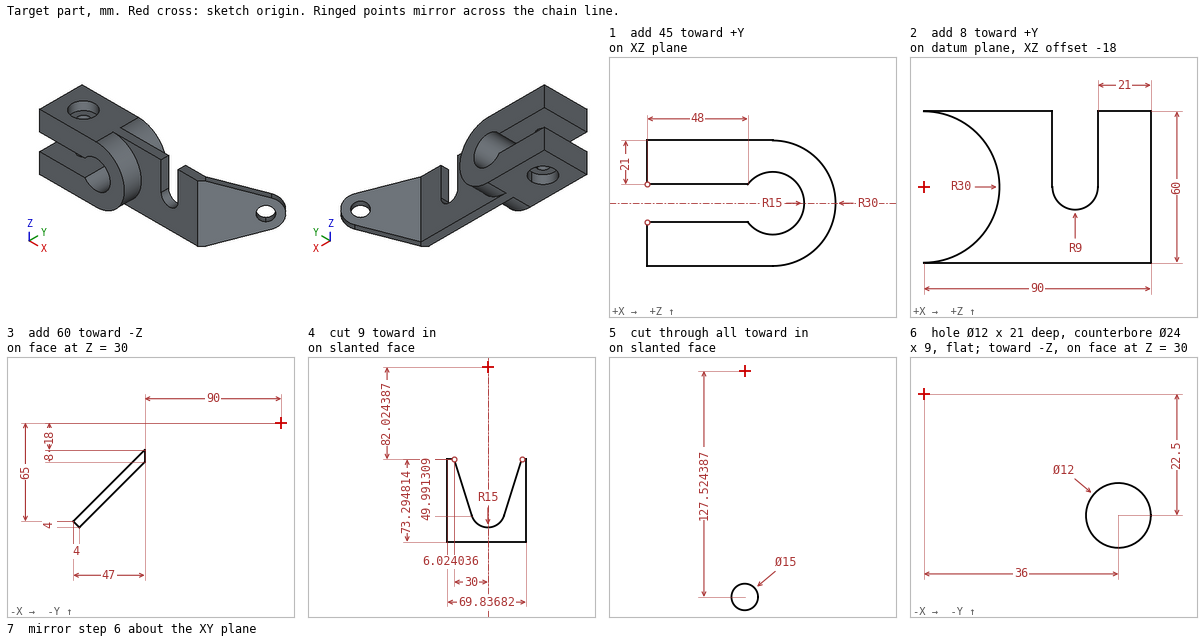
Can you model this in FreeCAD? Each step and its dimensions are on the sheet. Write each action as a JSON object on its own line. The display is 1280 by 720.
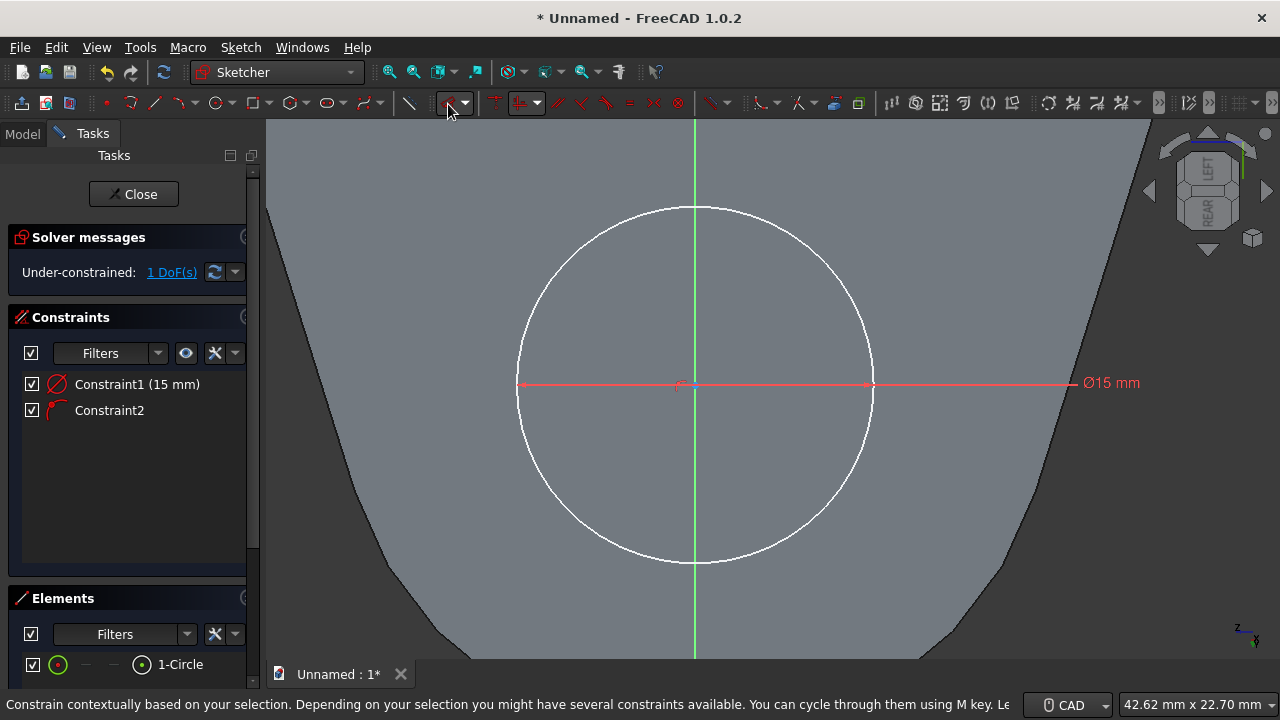
{"action": "left_click", "coordinate": [695, 385]}
{"action": "left_click", "coordinate": [729, 266]}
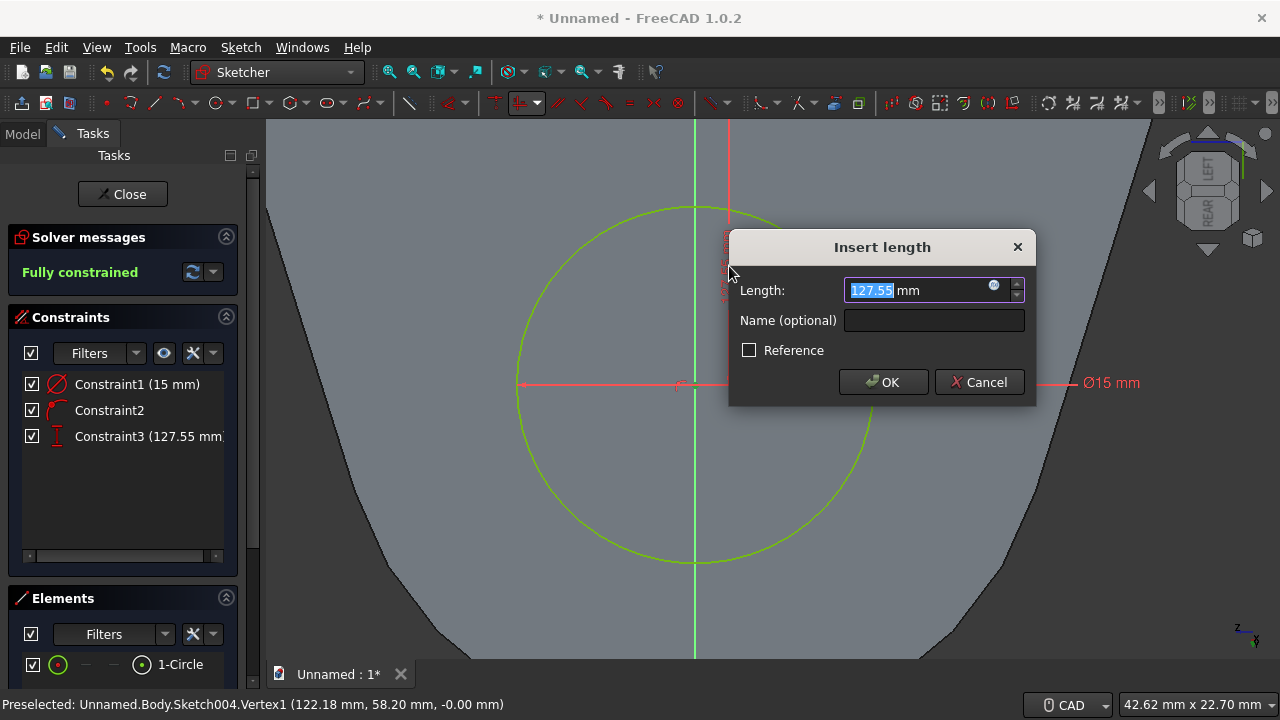
{"action": "type", "text": "127.524387"}
{"action": "key", "text": "Return"}
{"action": "key", "text": "Escape"}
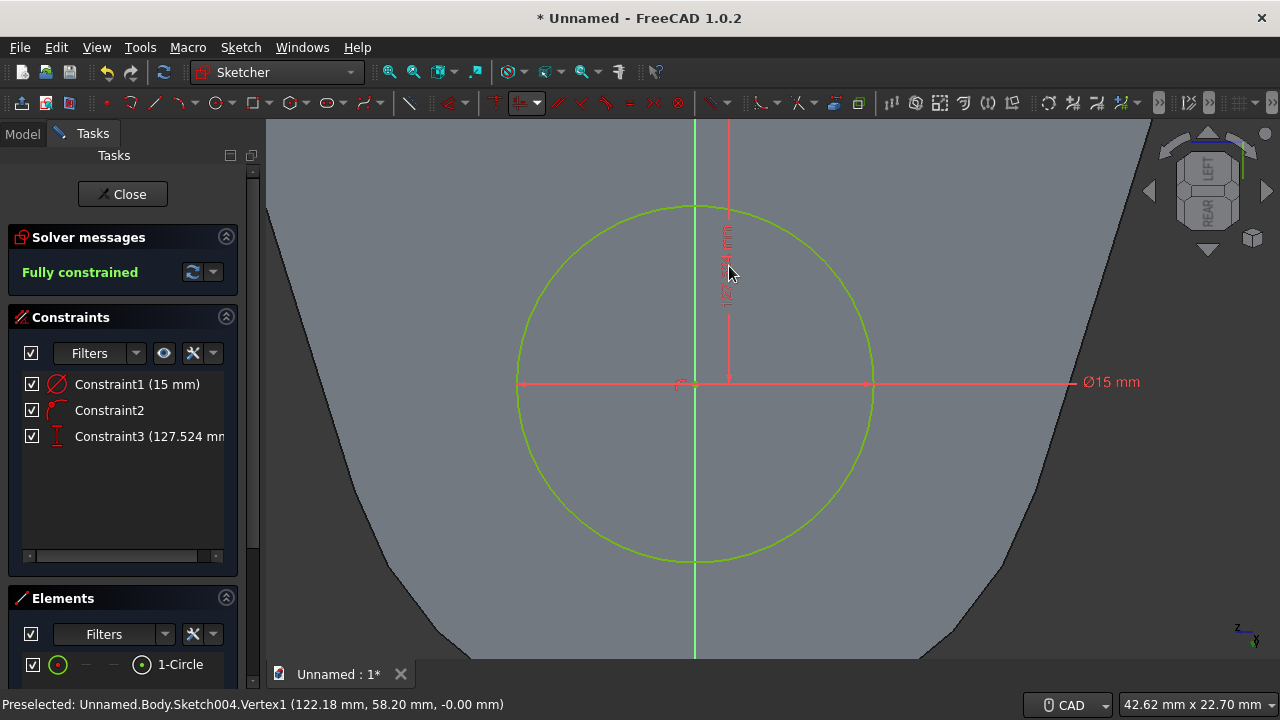
{"action": "left_click", "coordinate": [123, 194]}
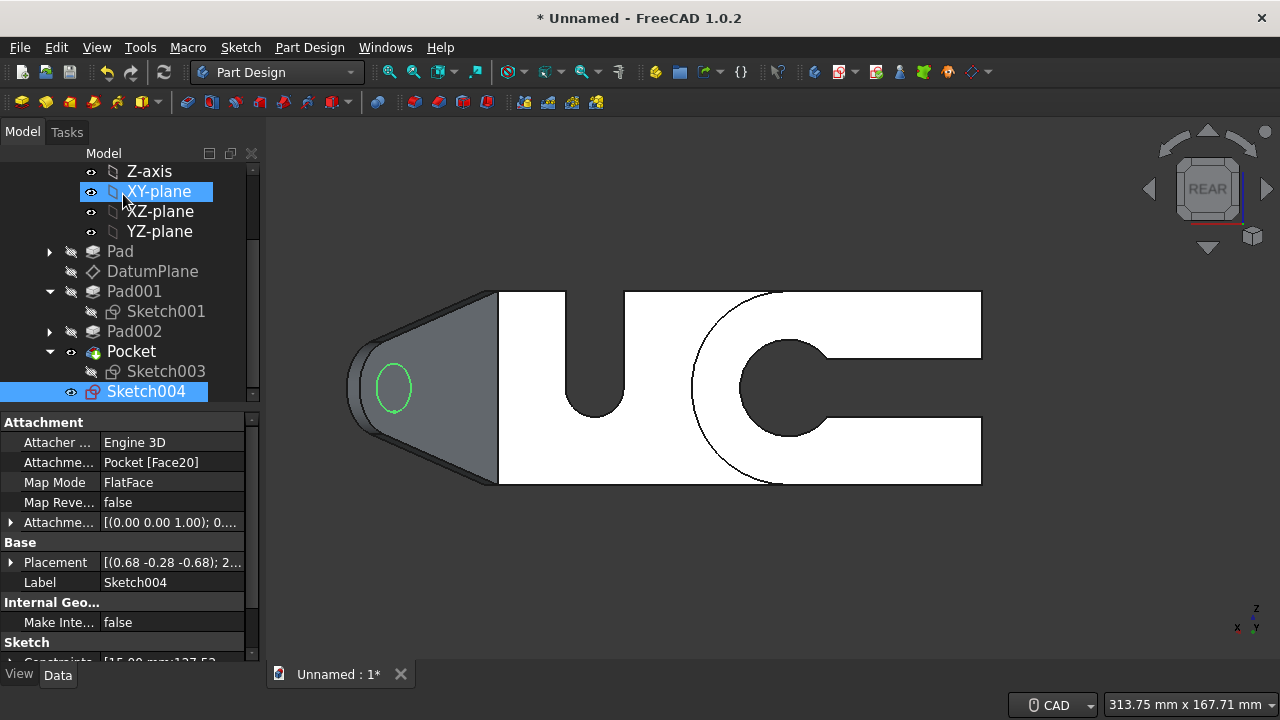
{"action": "left_click", "coordinate": [188, 102]}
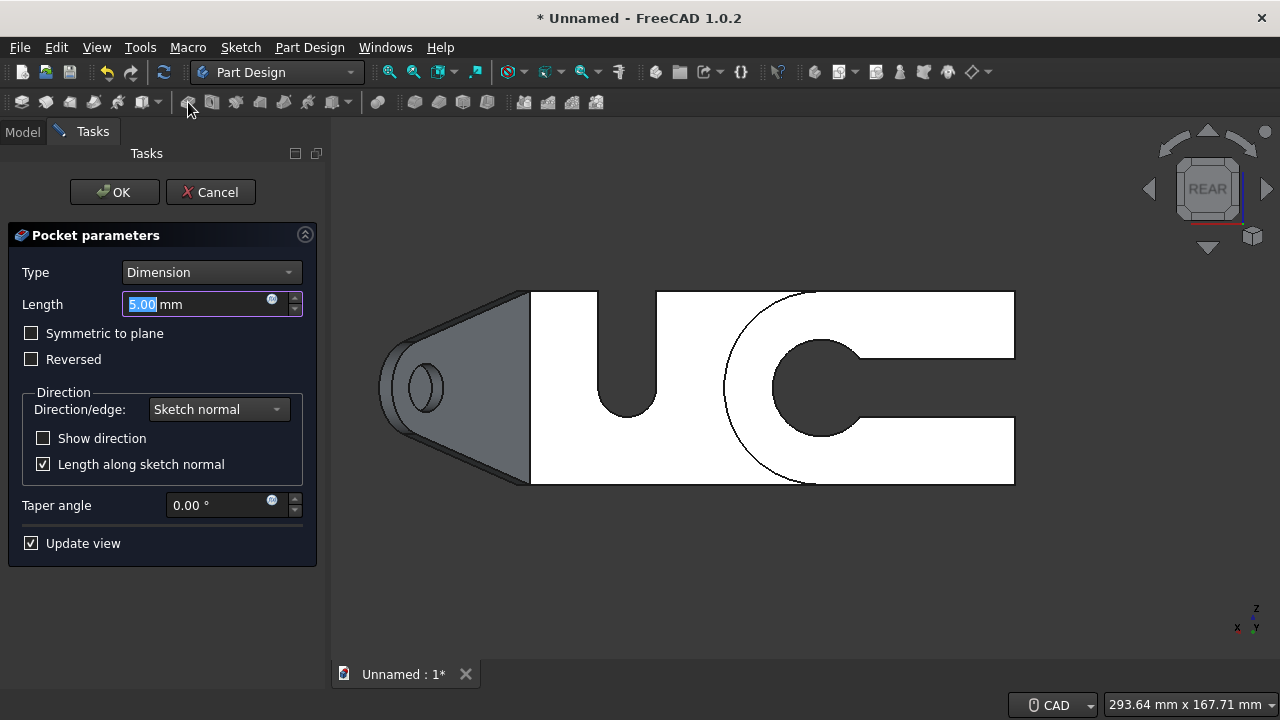
{"action": "left_click", "coordinate": [212, 272]}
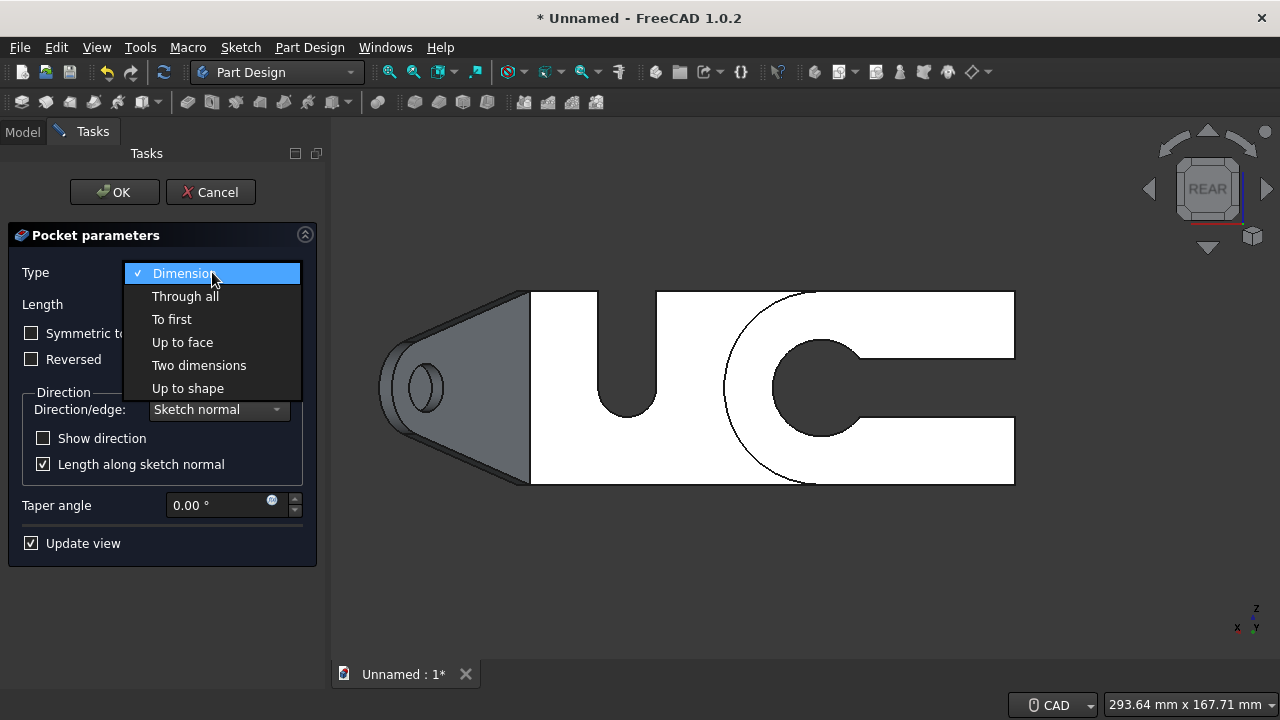
{"action": "left_click", "coordinate": [212, 296]}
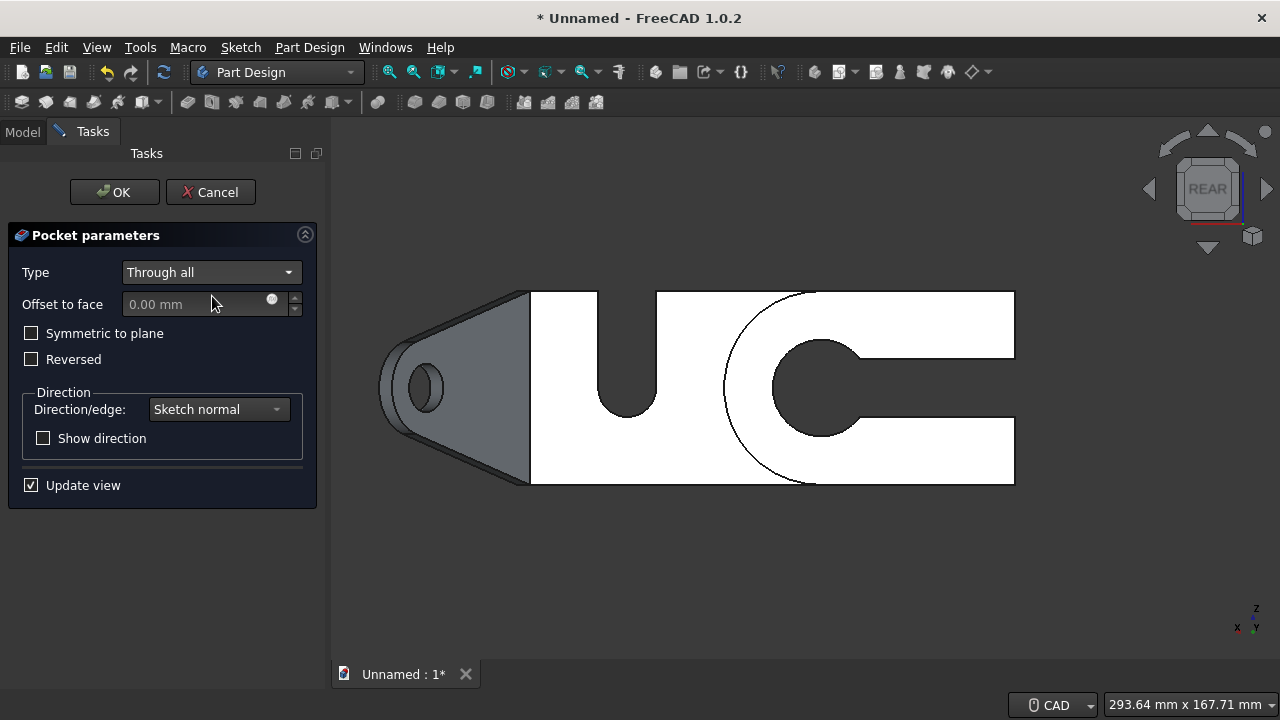
{"action": "left_click", "coordinate": [115, 192]}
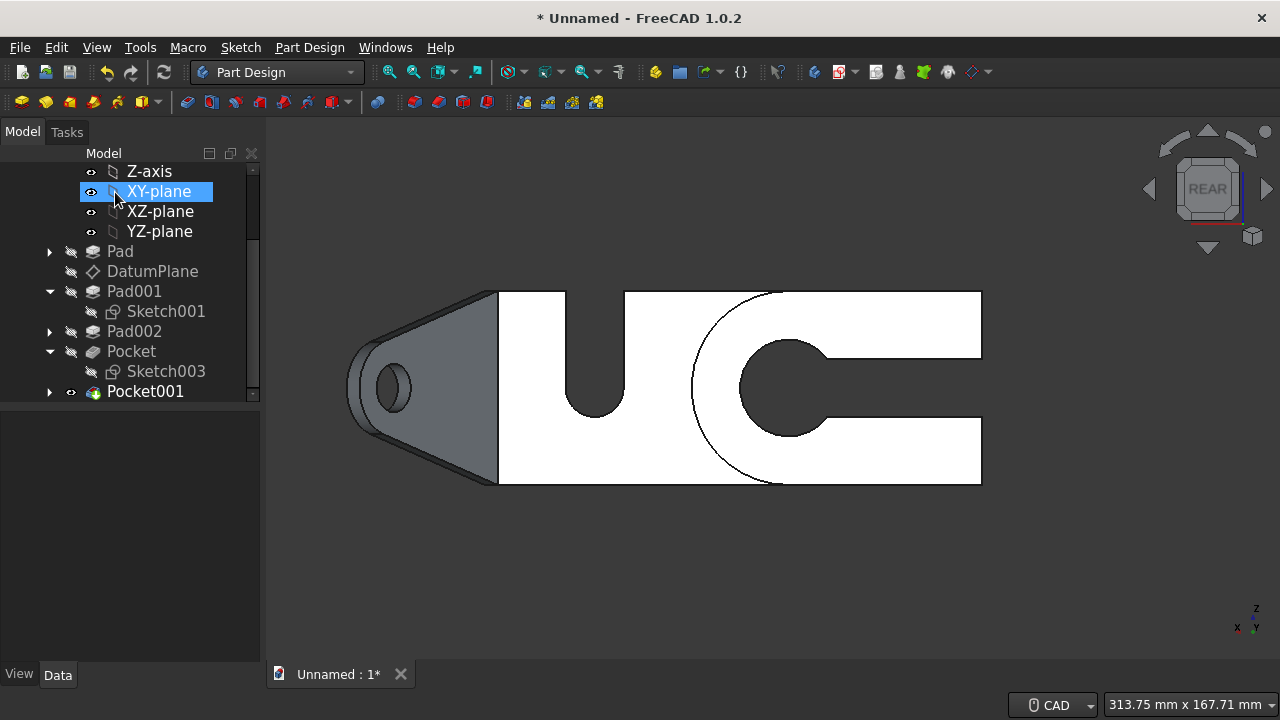
{"action": "key", "text": "0"}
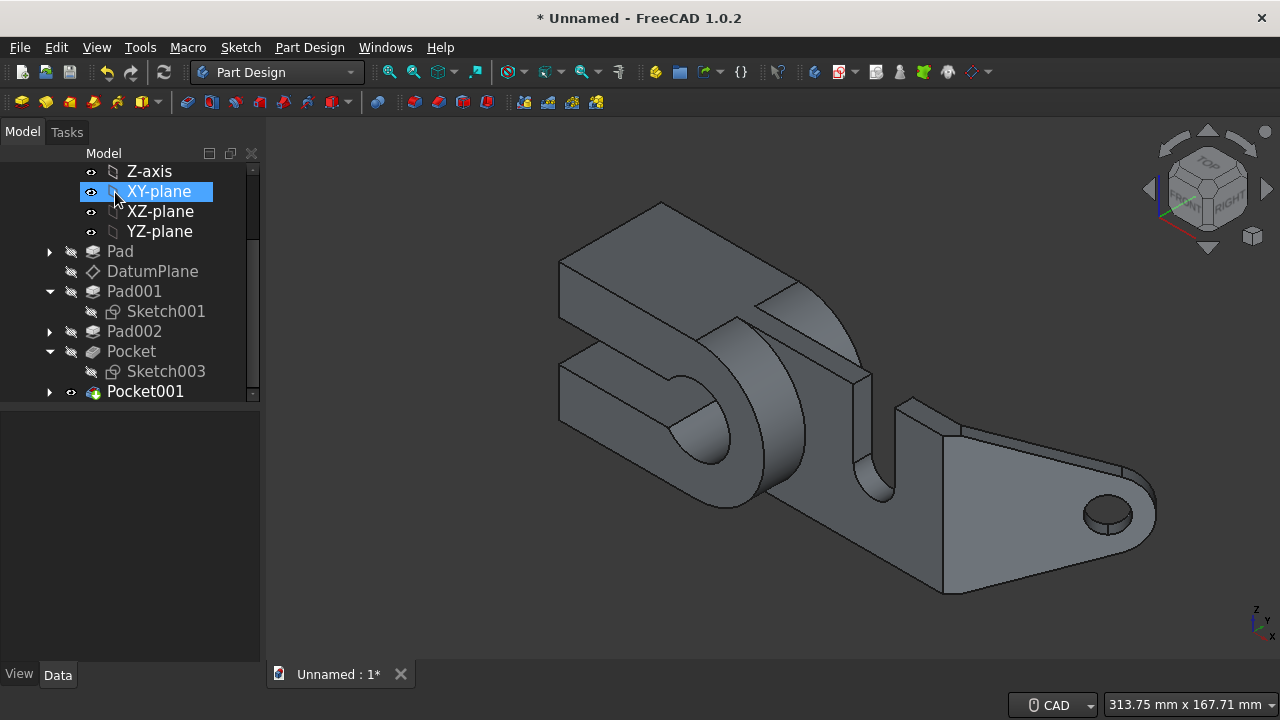
{"action": "key", "text": "v f"}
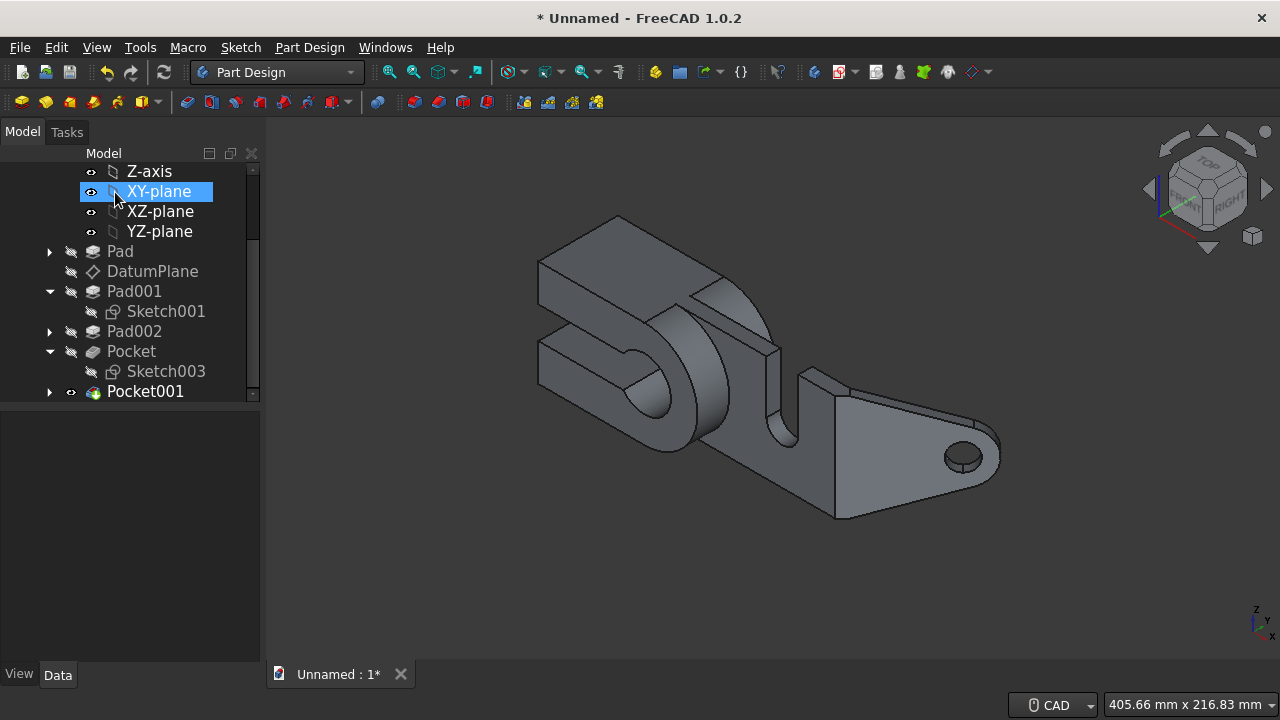
{"action": "left_click", "coordinate": [620, 262]}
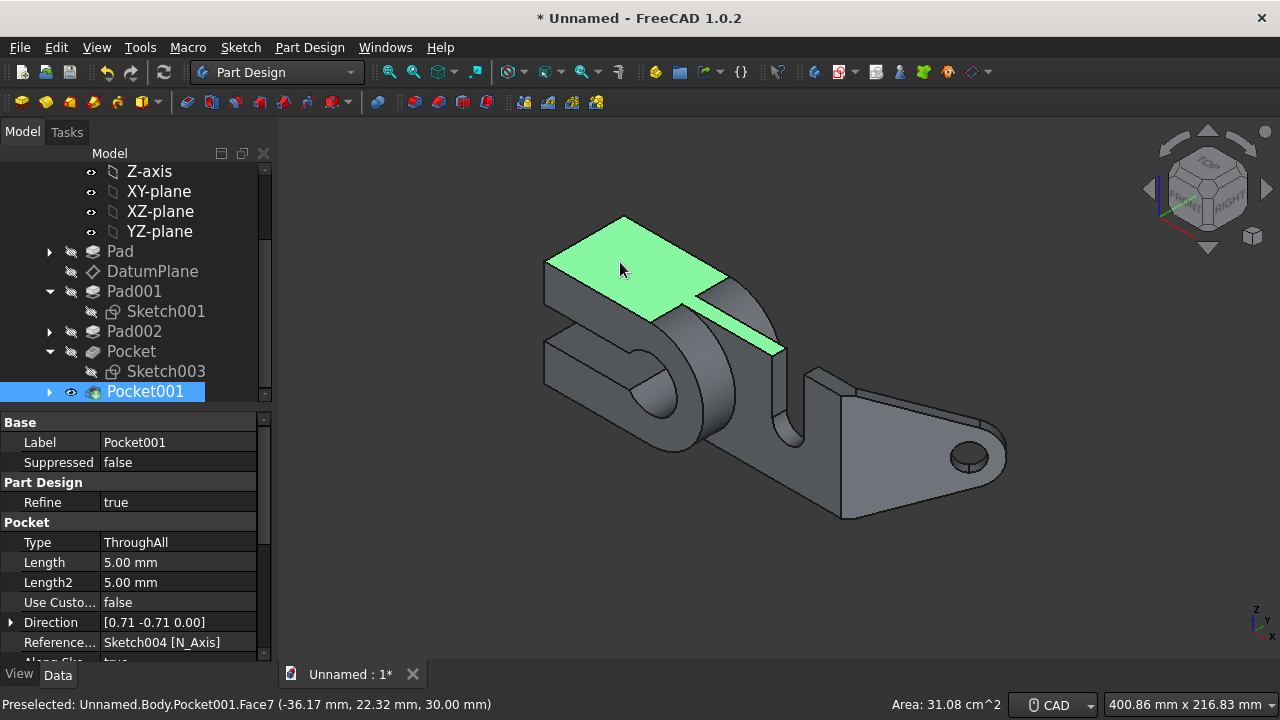
{"action": "left_click", "coordinate": [840, 72]}